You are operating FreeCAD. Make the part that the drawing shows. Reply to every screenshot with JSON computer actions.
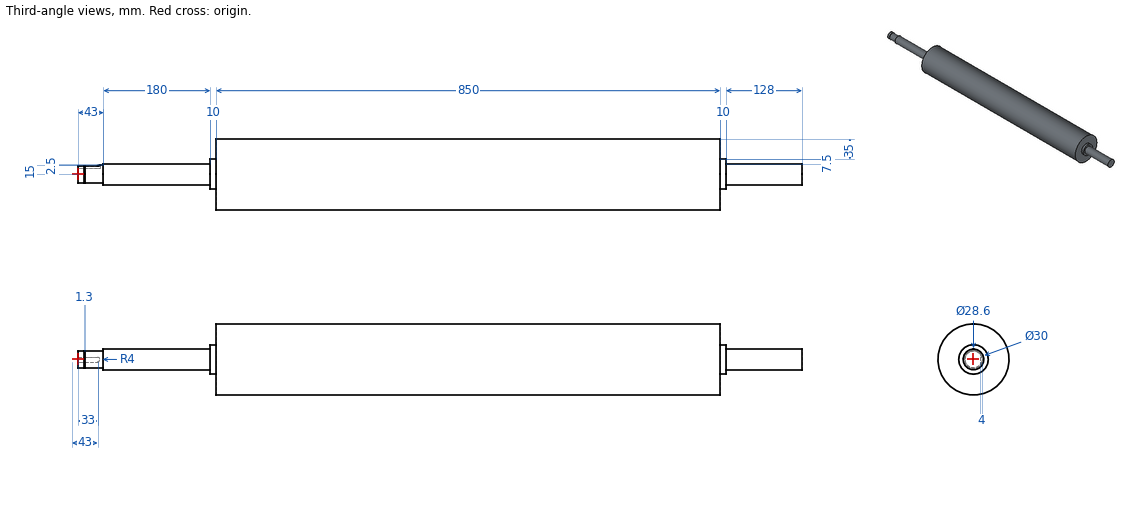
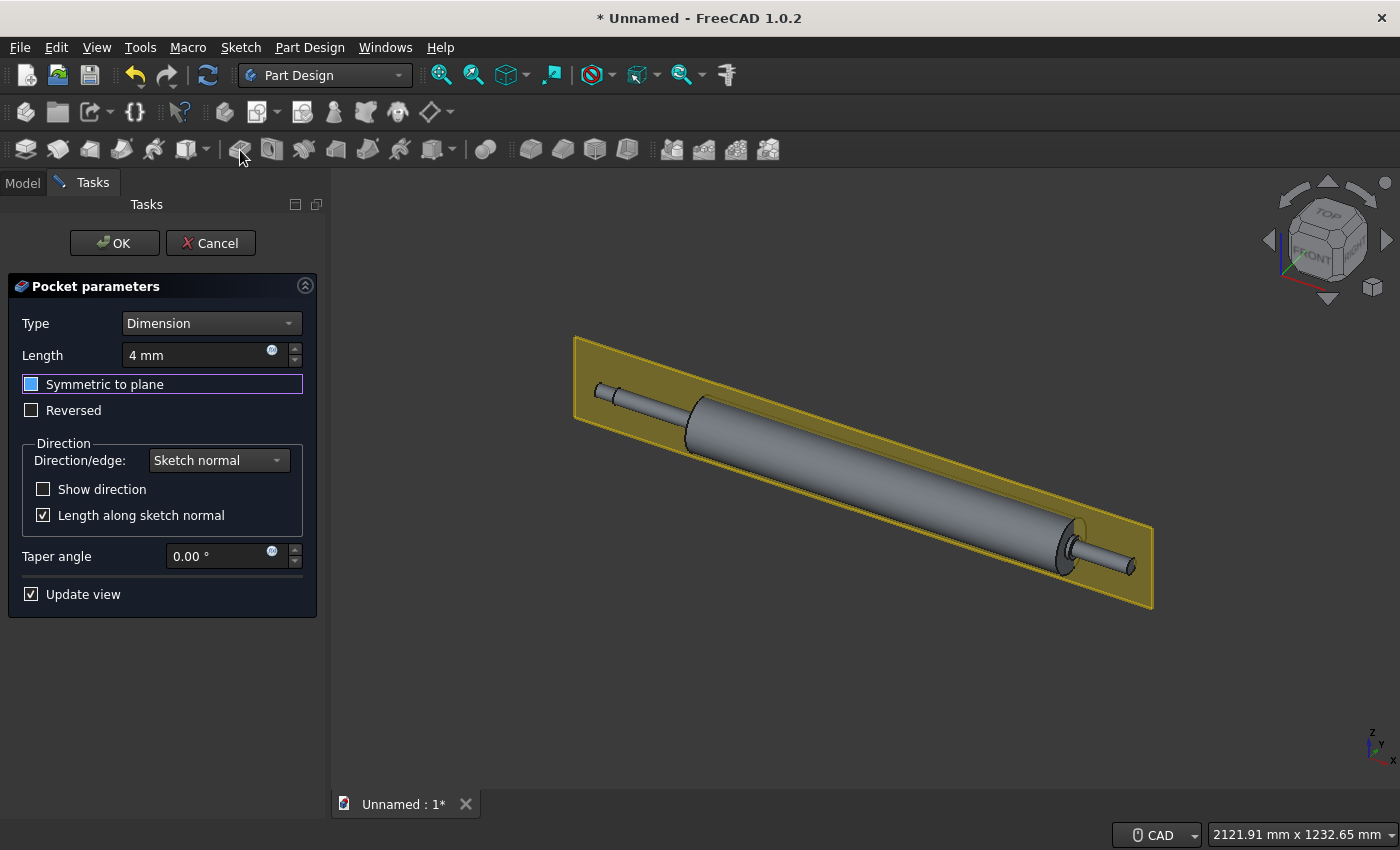
{"action": "left_click", "coordinate": [30, 410]}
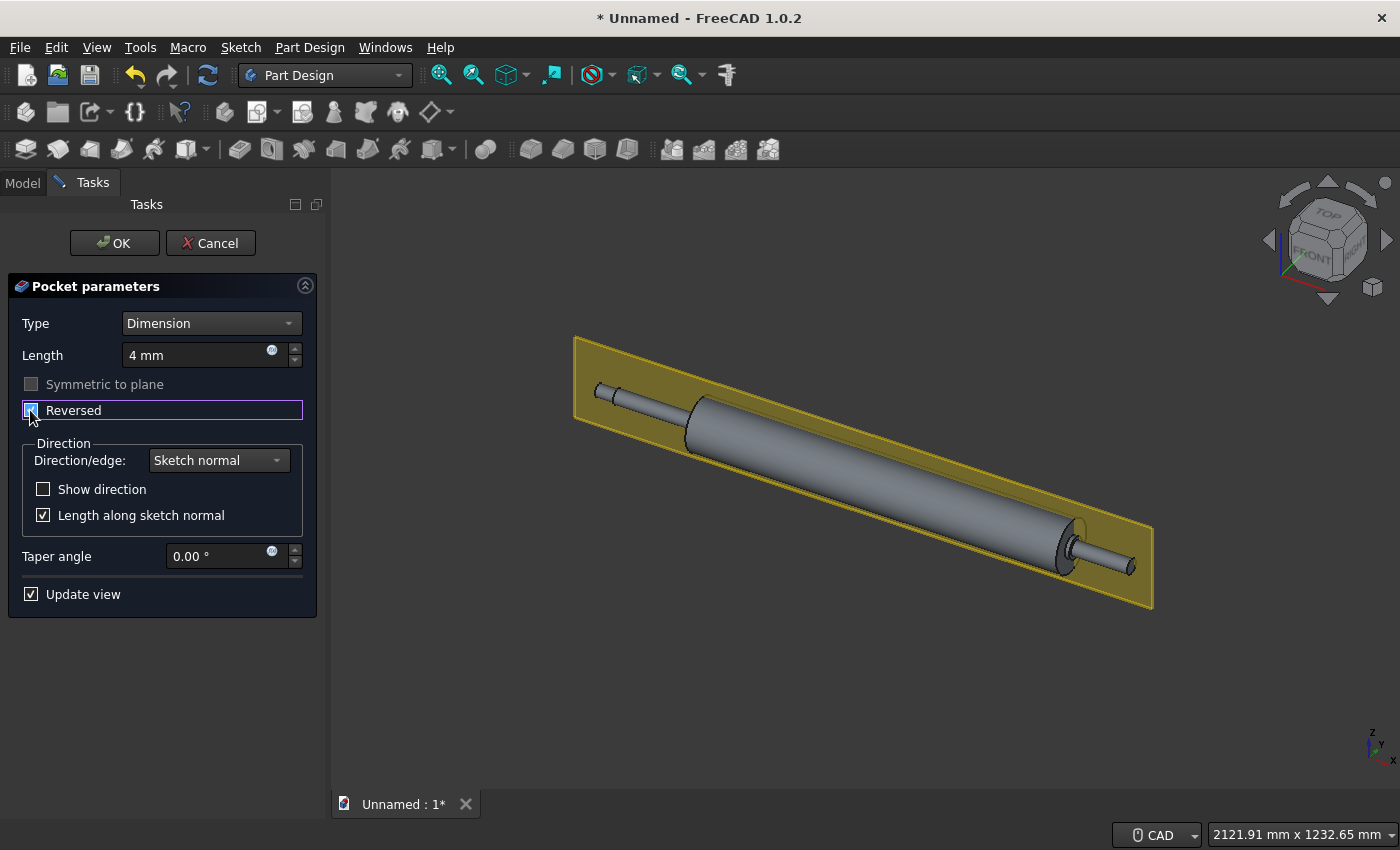
{"action": "left_click", "coordinate": [115, 243]}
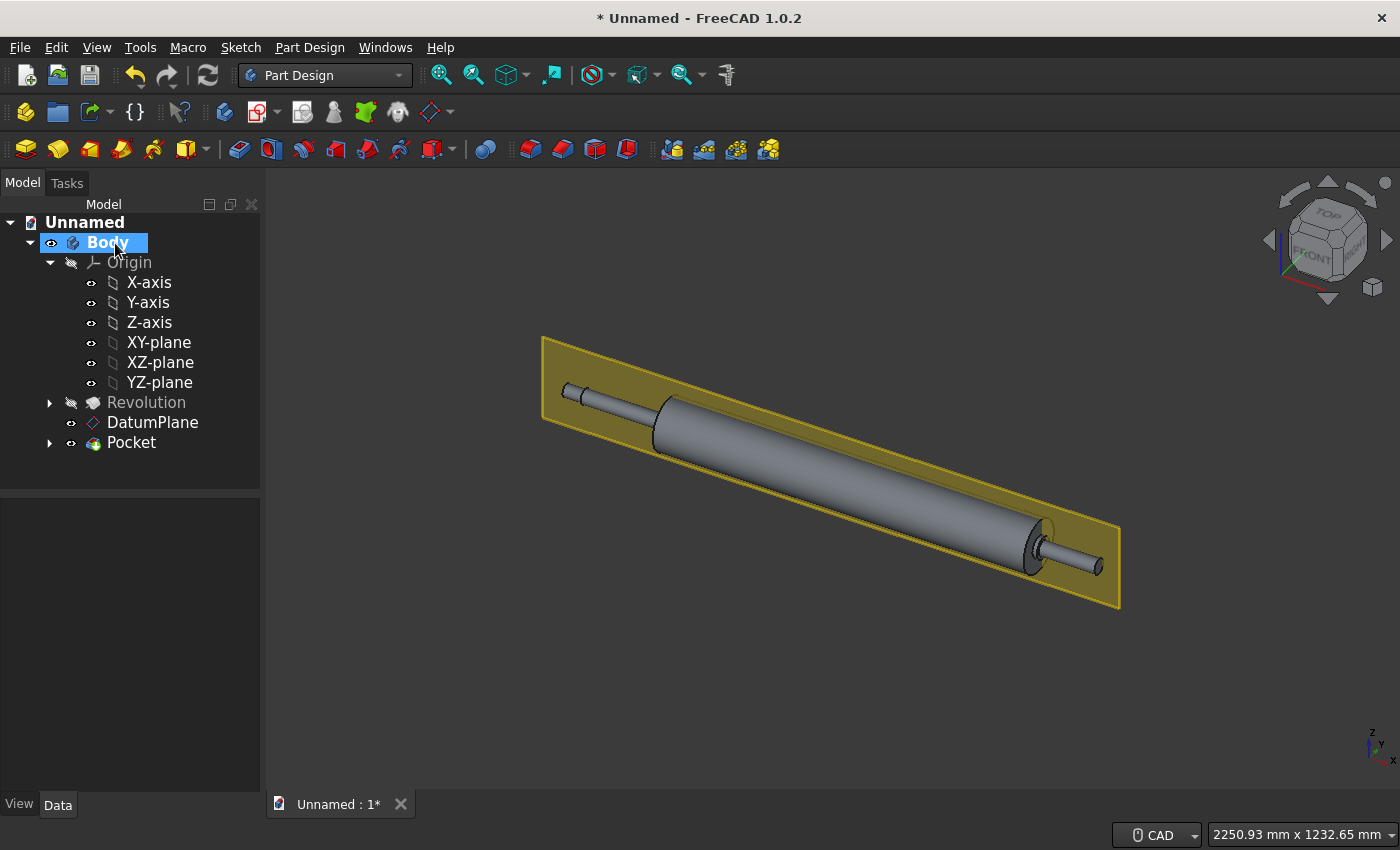
{"action": "left_click", "coordinate": [116, 423]}
{"action": "key", "text": "space"}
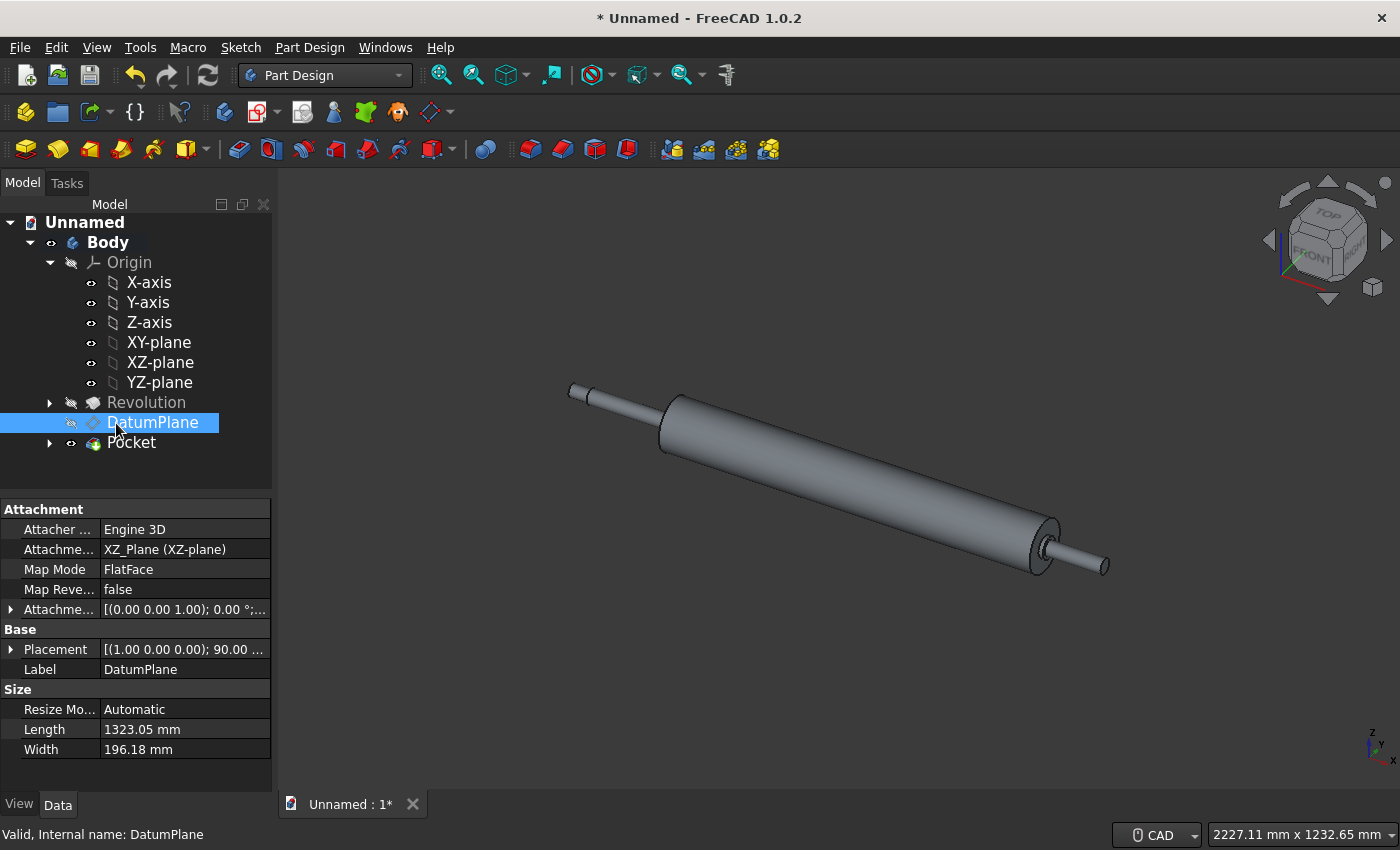
{"action": "left_click", "coordinate": [136, 383]}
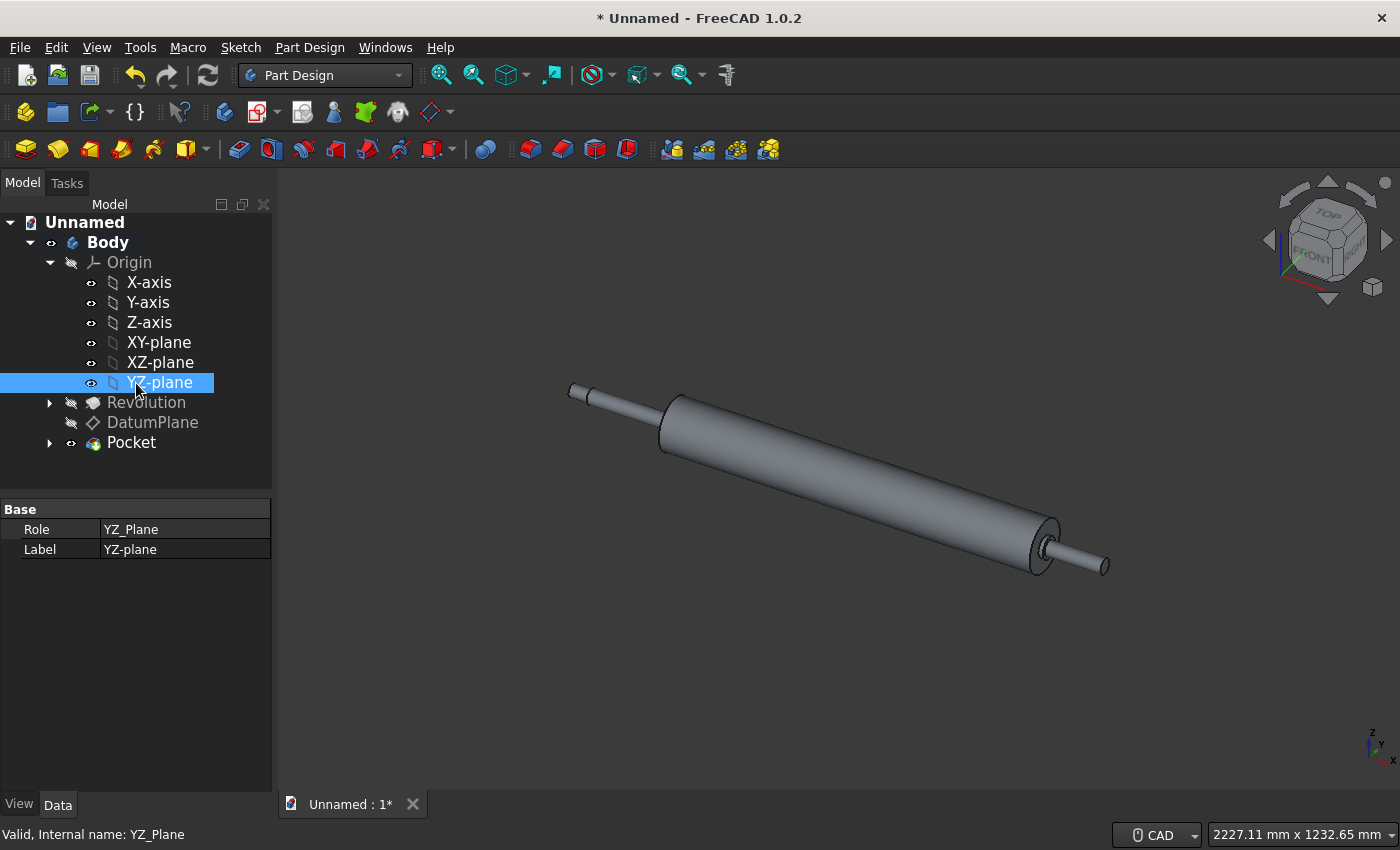
{"action": "left_click", "coordinate": [430, 112]}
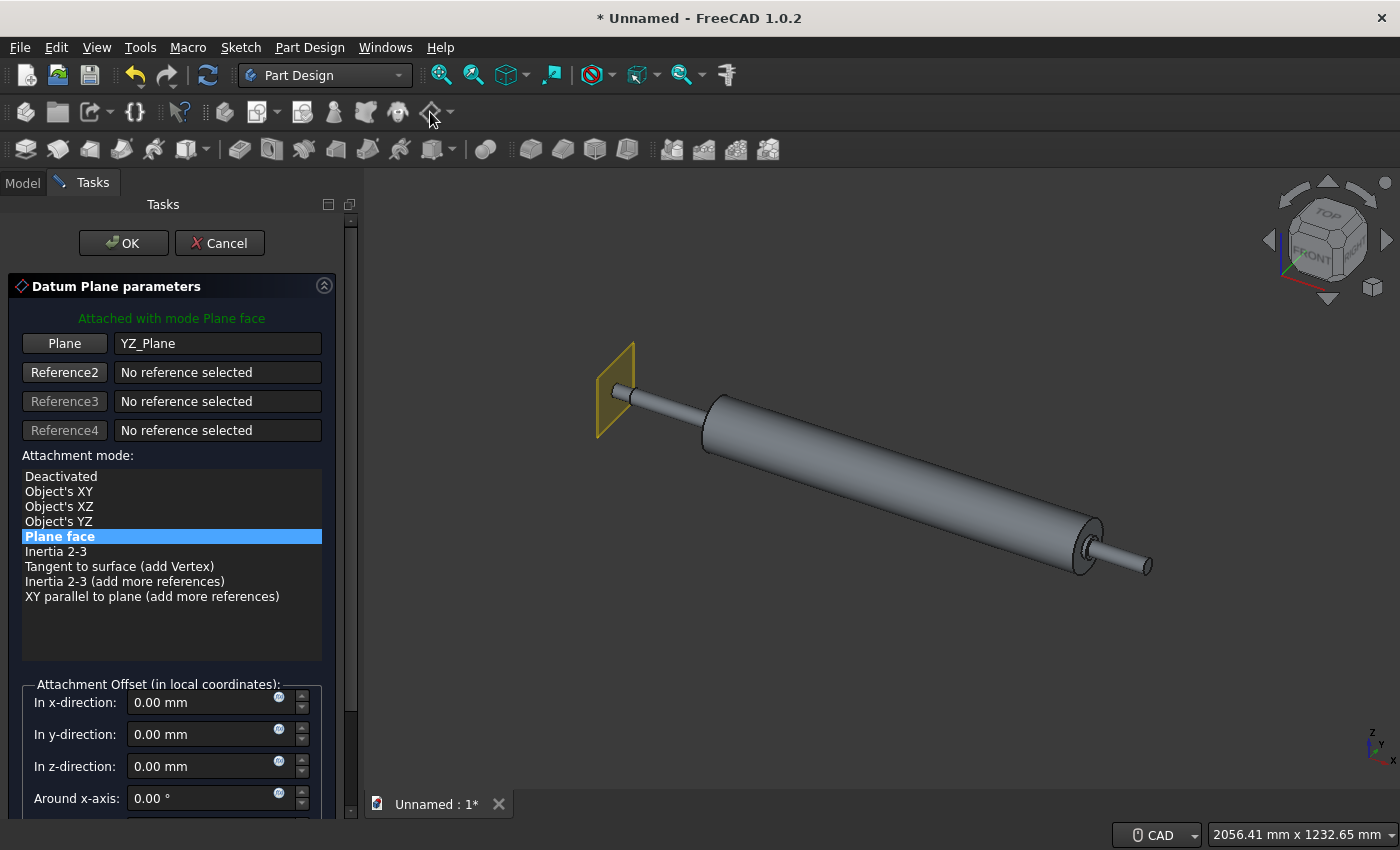
{"action": "triple_click", "coordinate": [210, 766]}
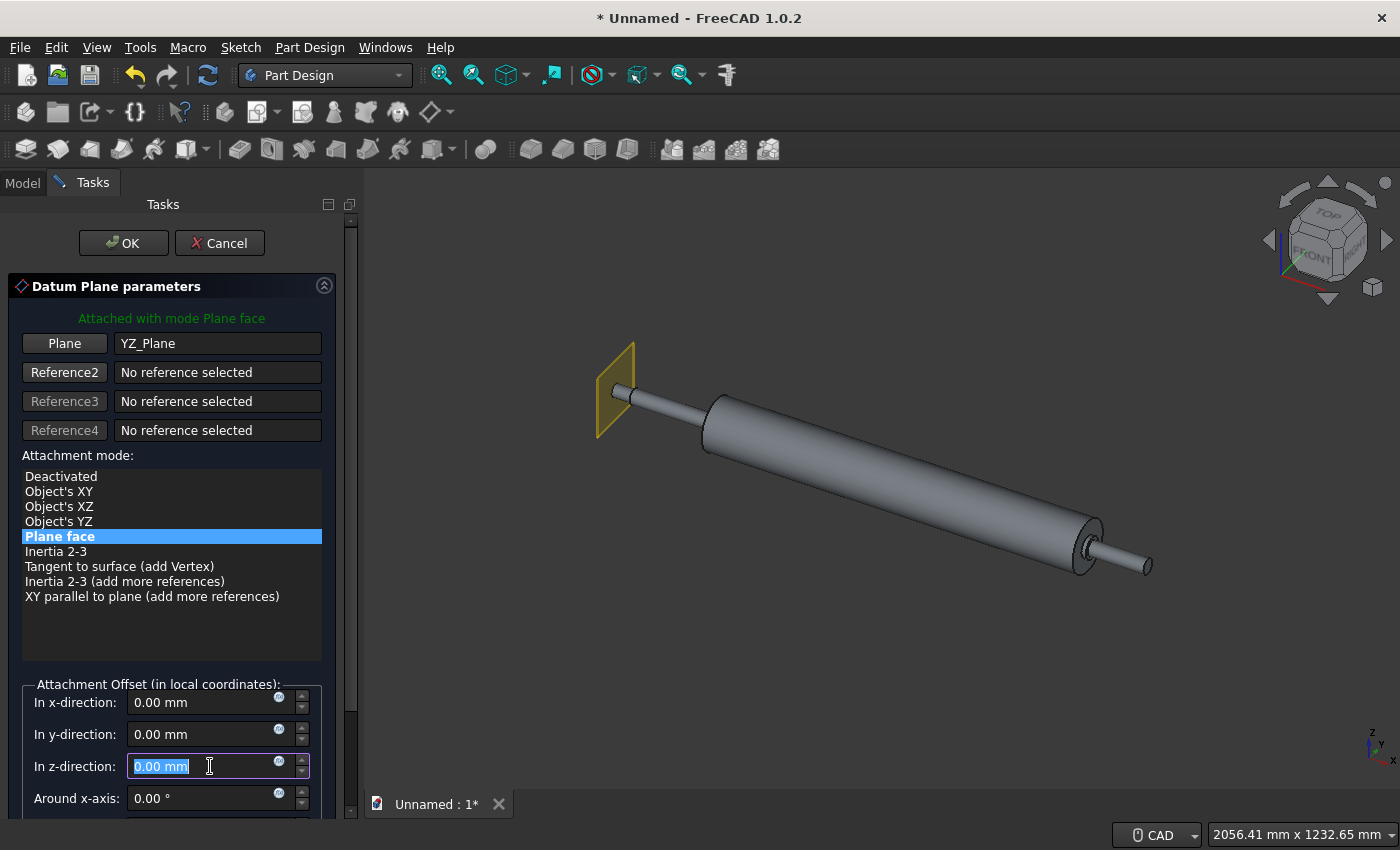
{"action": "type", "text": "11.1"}
{"action": "key", "text": "Tab"}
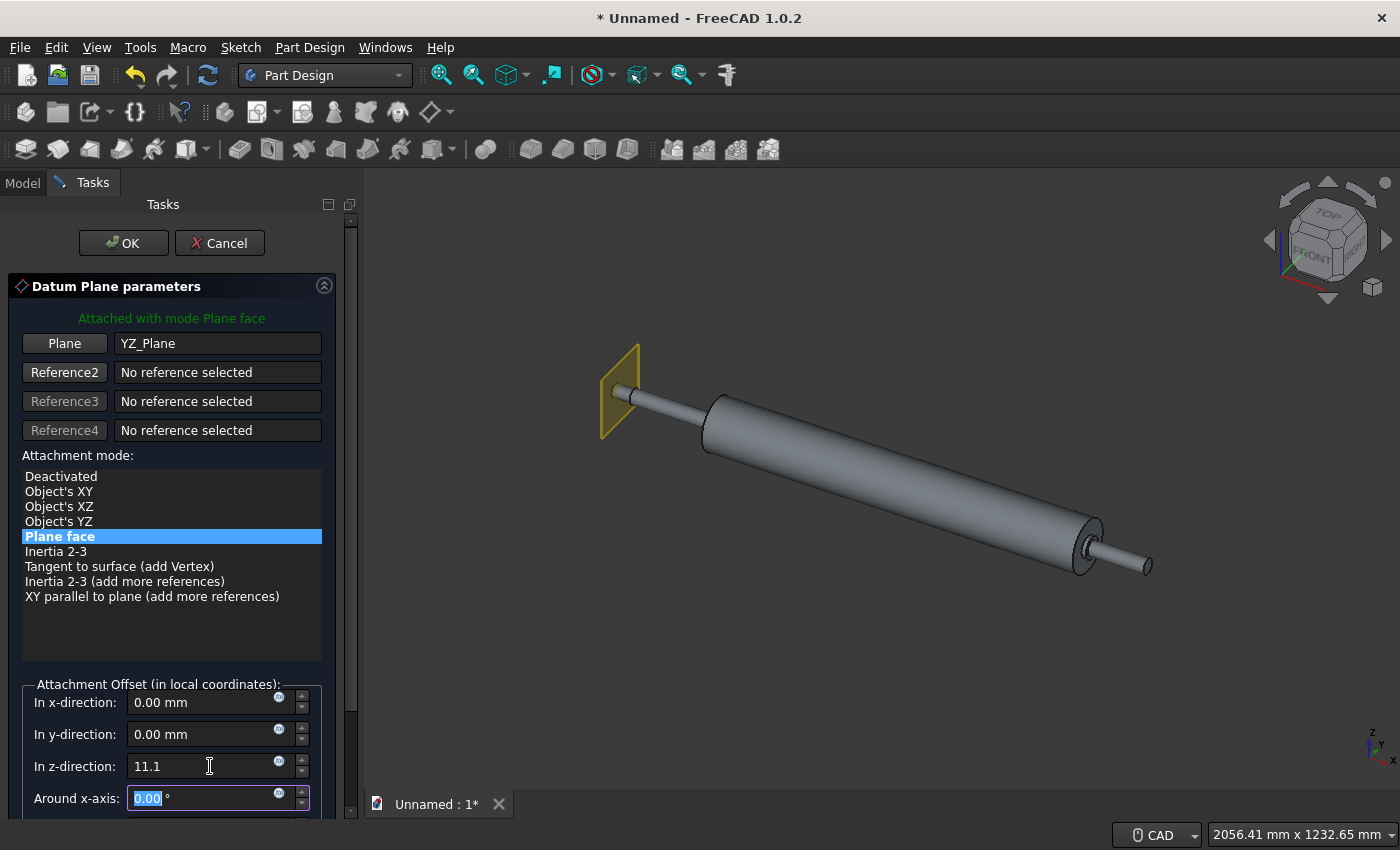
{"action": "left_click", "coordinate": [124, 243]}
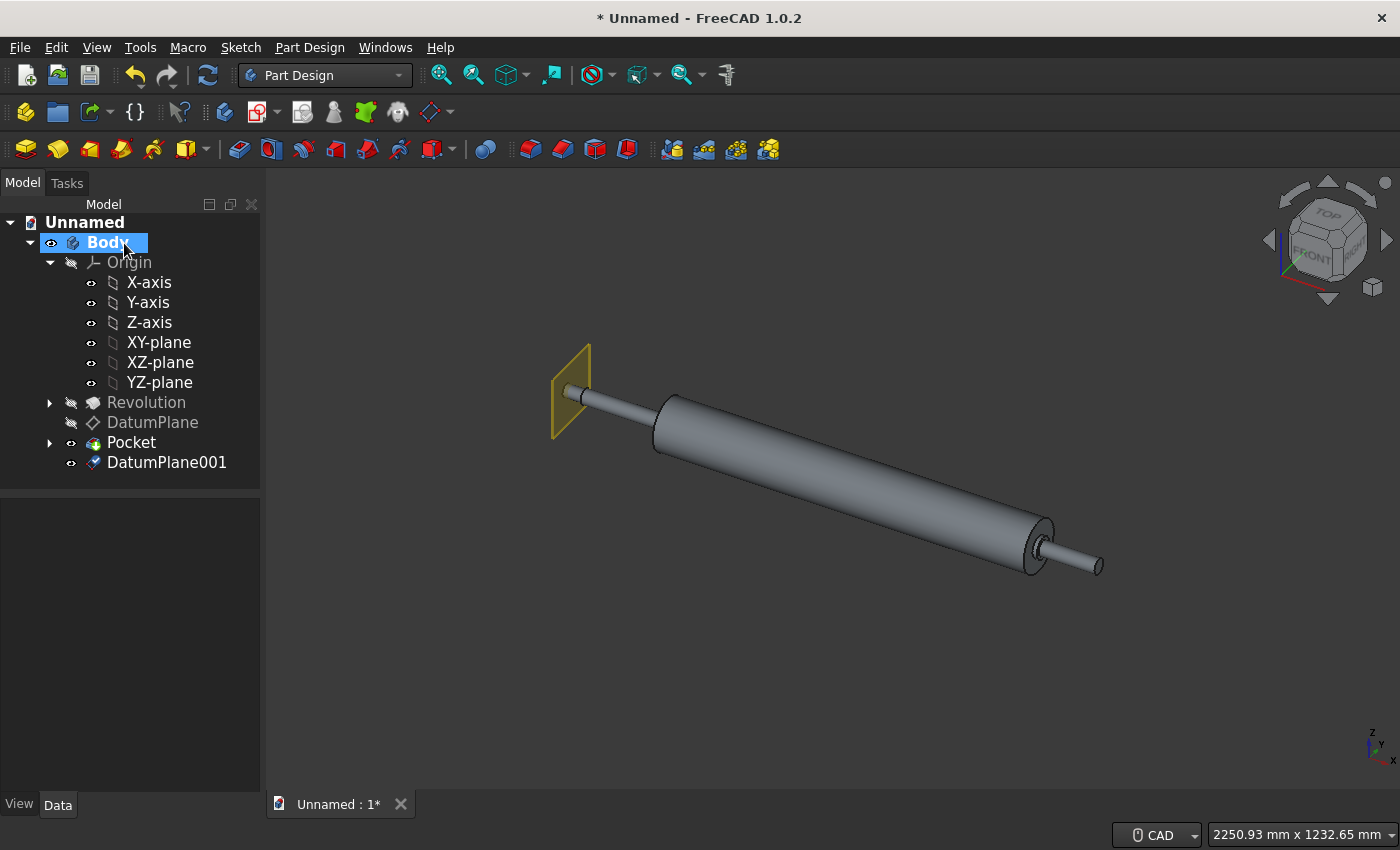
{"action": "left_click", "coordinate": [116, 463]}